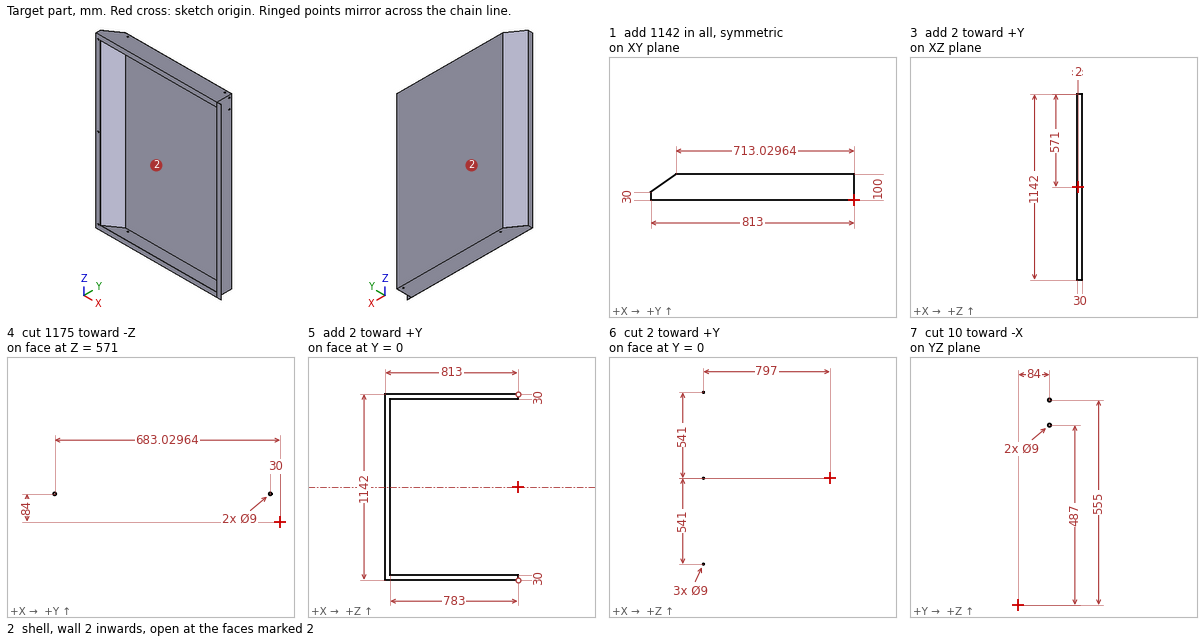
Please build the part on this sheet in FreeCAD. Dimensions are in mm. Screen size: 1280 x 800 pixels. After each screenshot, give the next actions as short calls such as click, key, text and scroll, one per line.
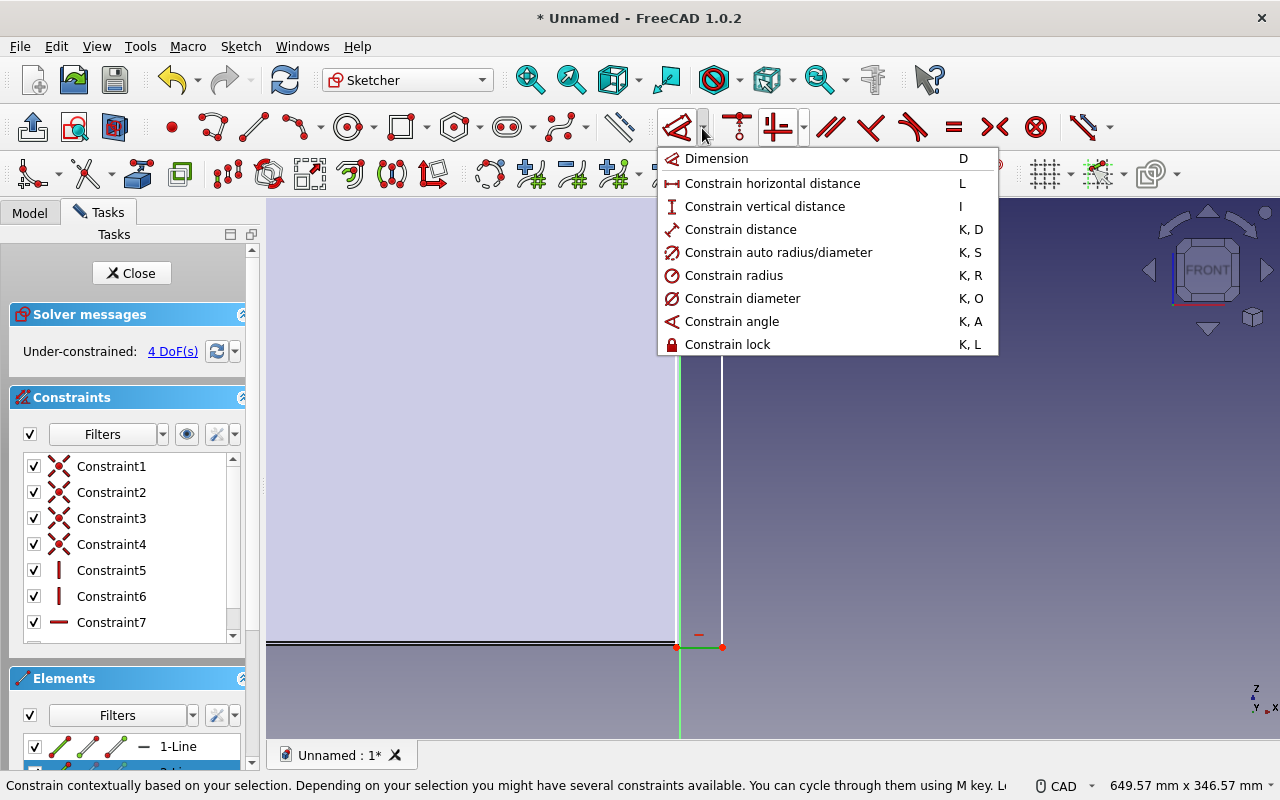
click(828, 184)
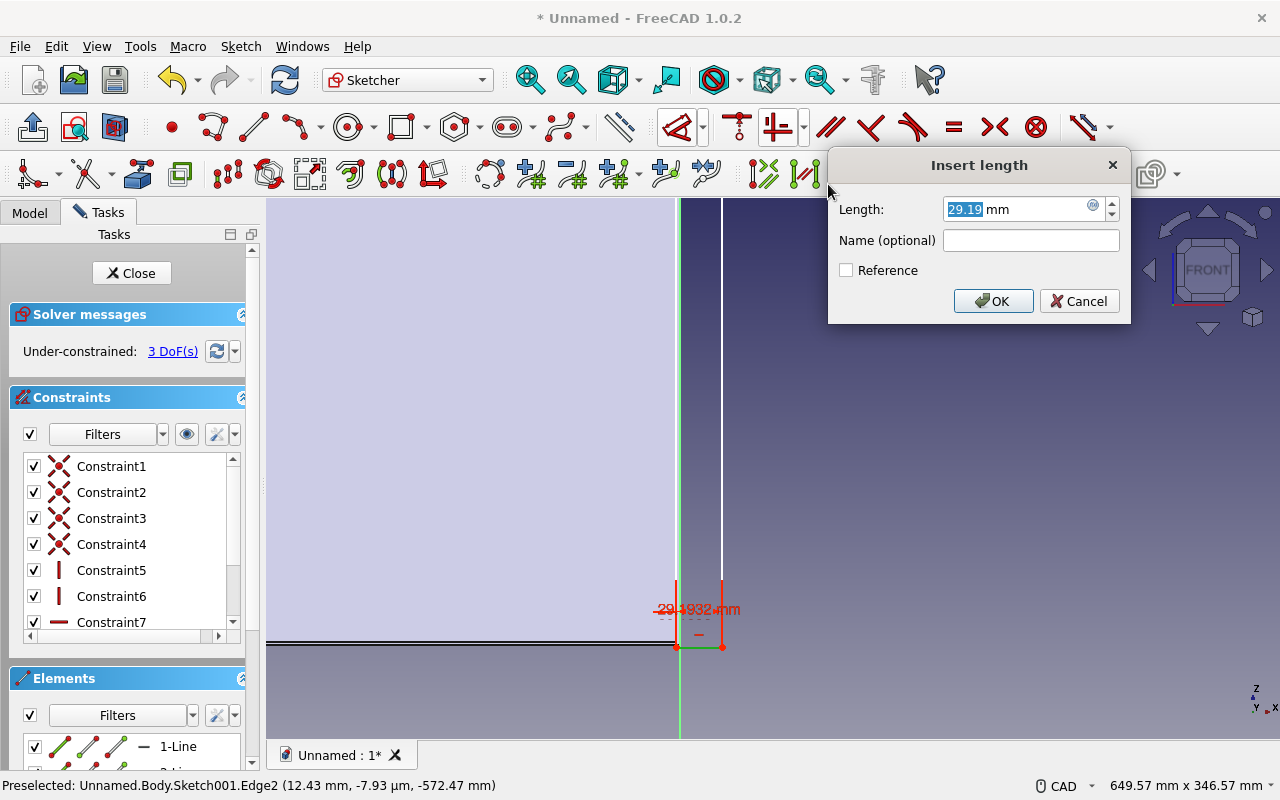
text(30)
key(Return)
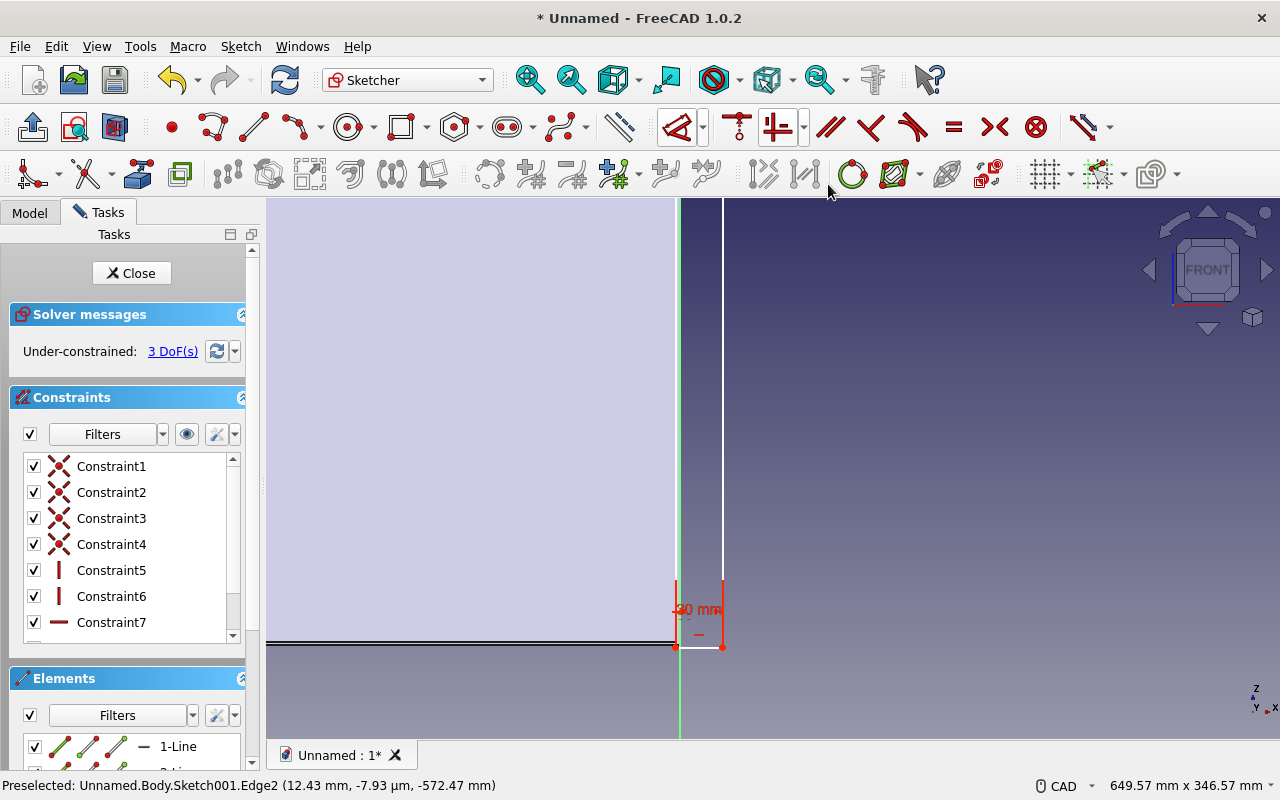
scroll(706, 649, down, 8)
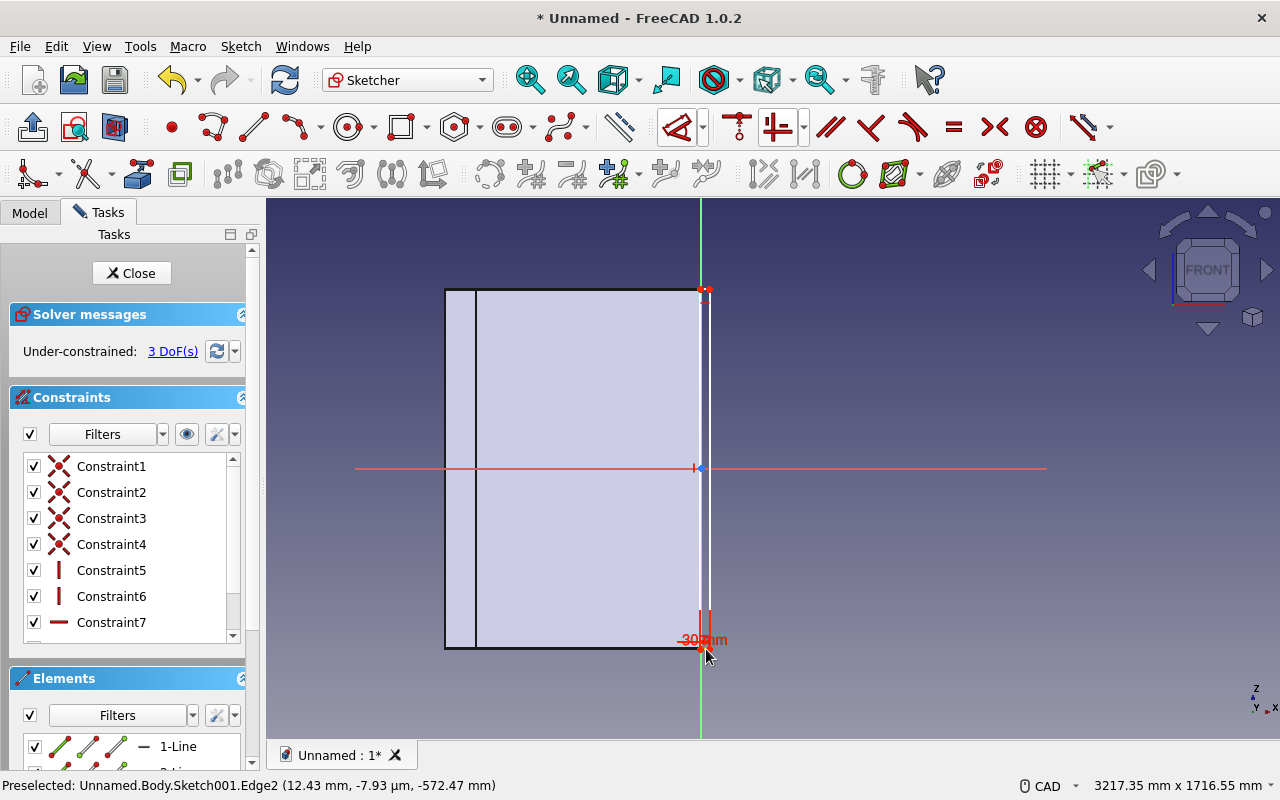
scroll(700, 289, up, 21)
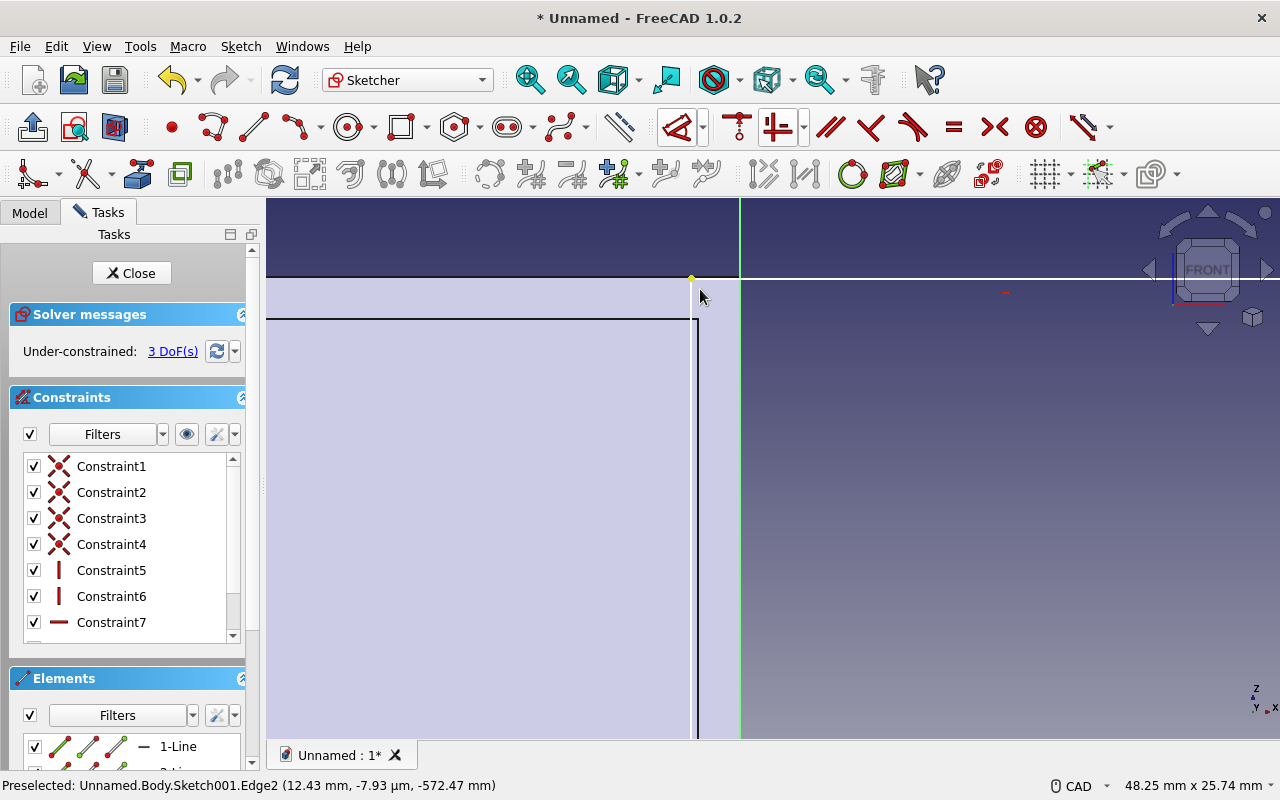
click(691, 279)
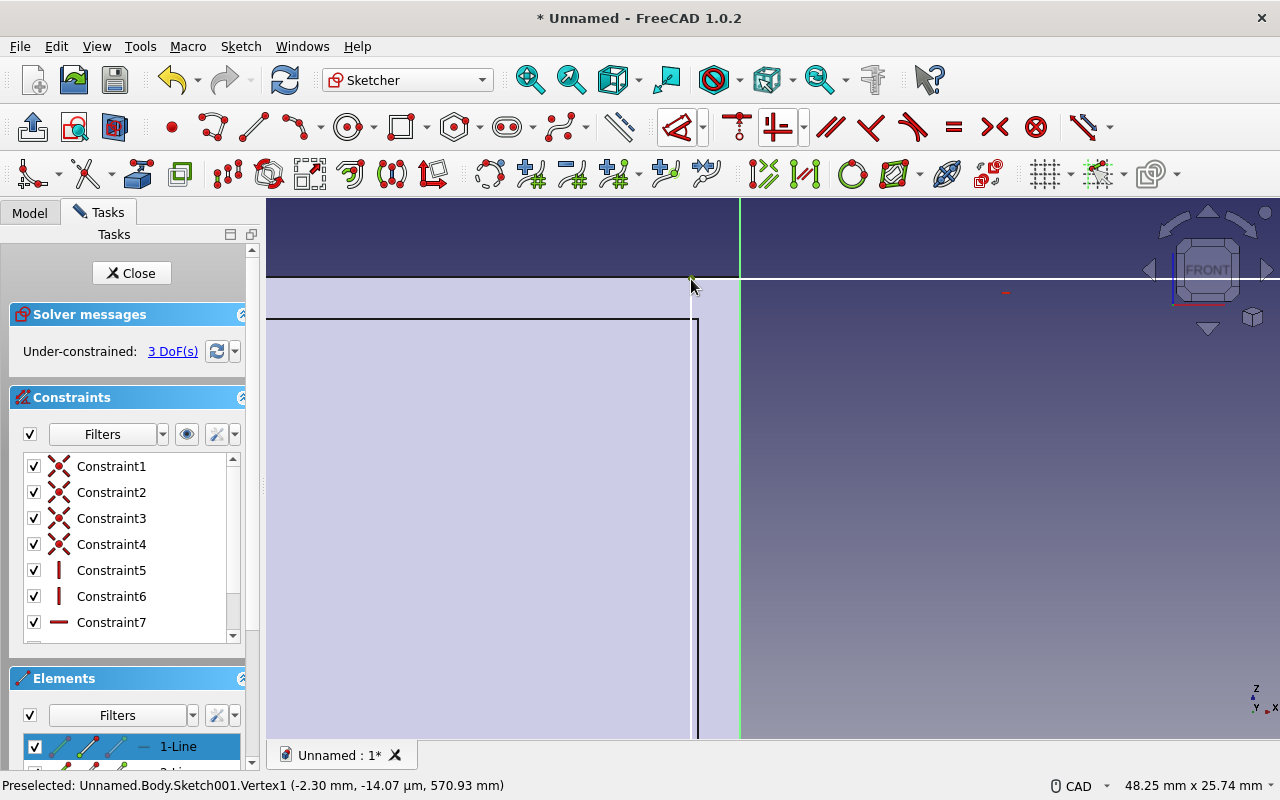
key(l)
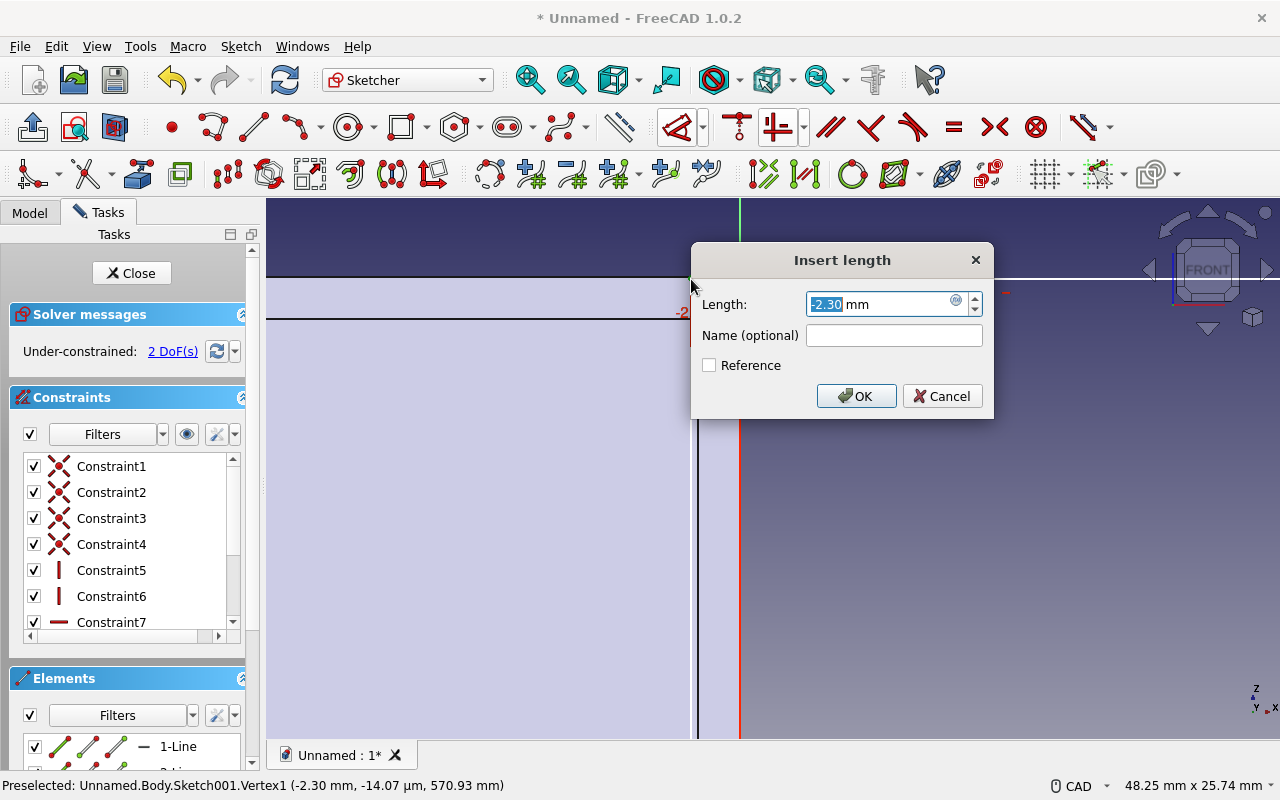
text(-2)
key(Return)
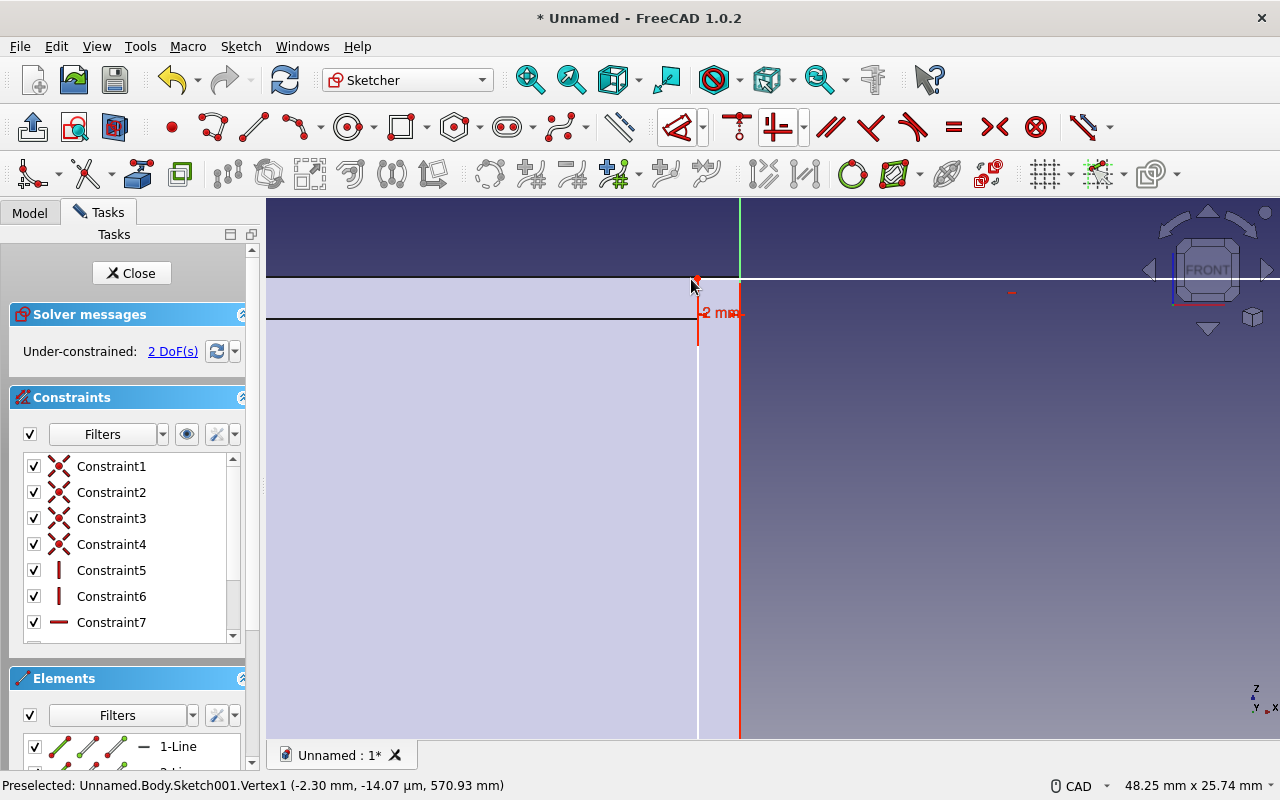
scroll(704, 468, down, 15)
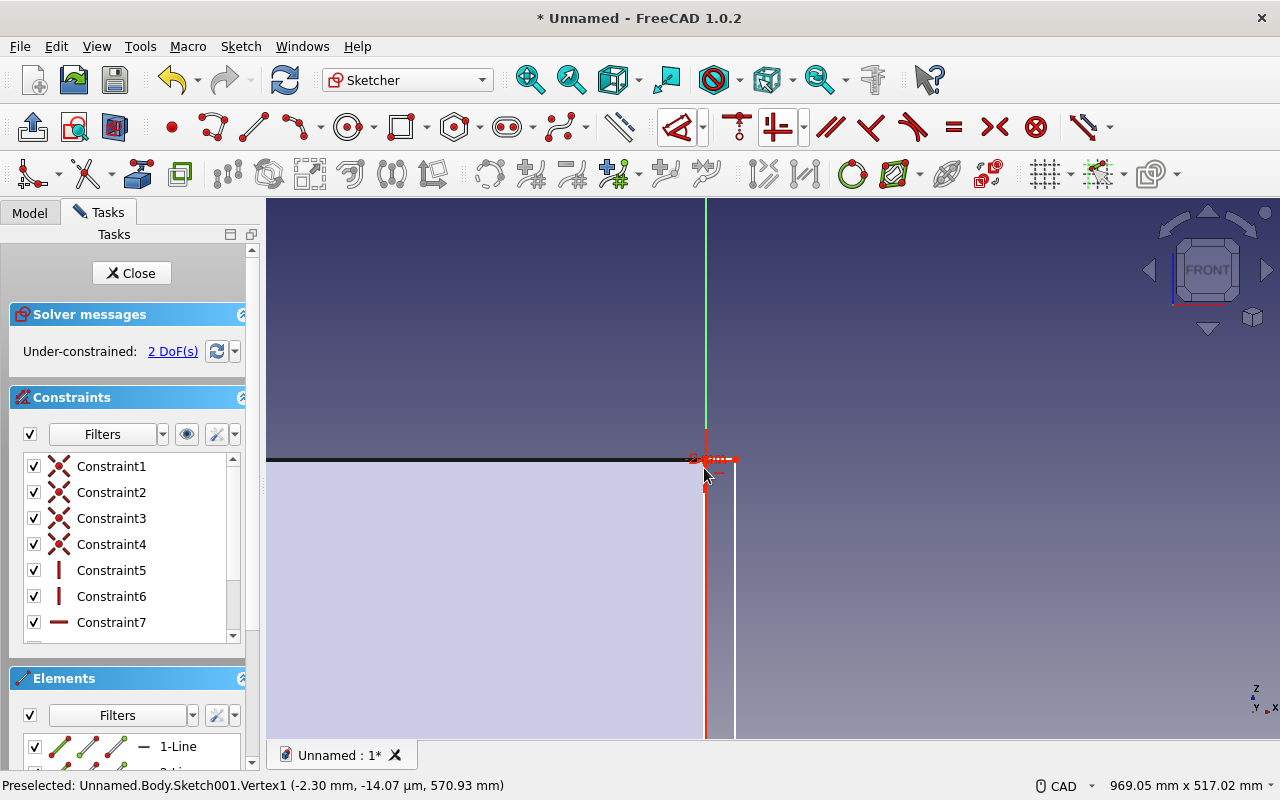
scroll(698, 226, down, 6)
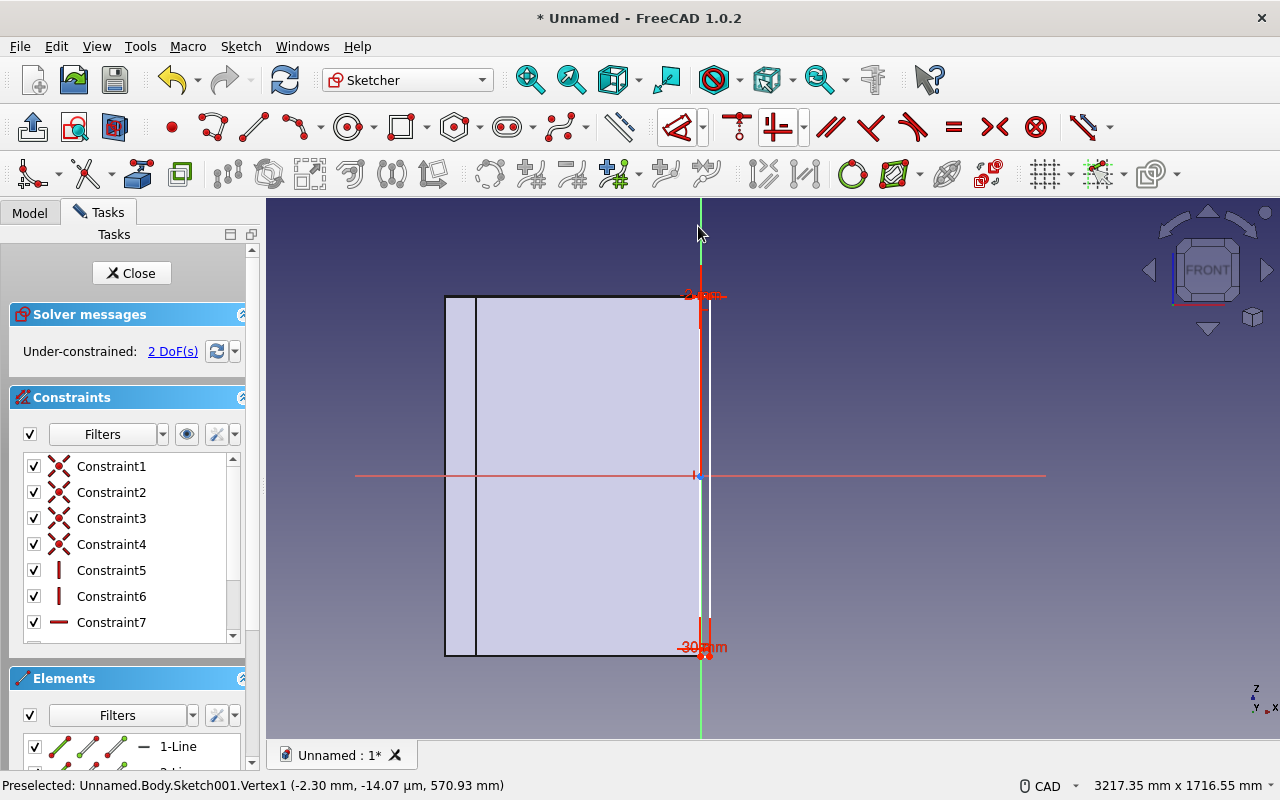
scroll(700, 404, up, 14)